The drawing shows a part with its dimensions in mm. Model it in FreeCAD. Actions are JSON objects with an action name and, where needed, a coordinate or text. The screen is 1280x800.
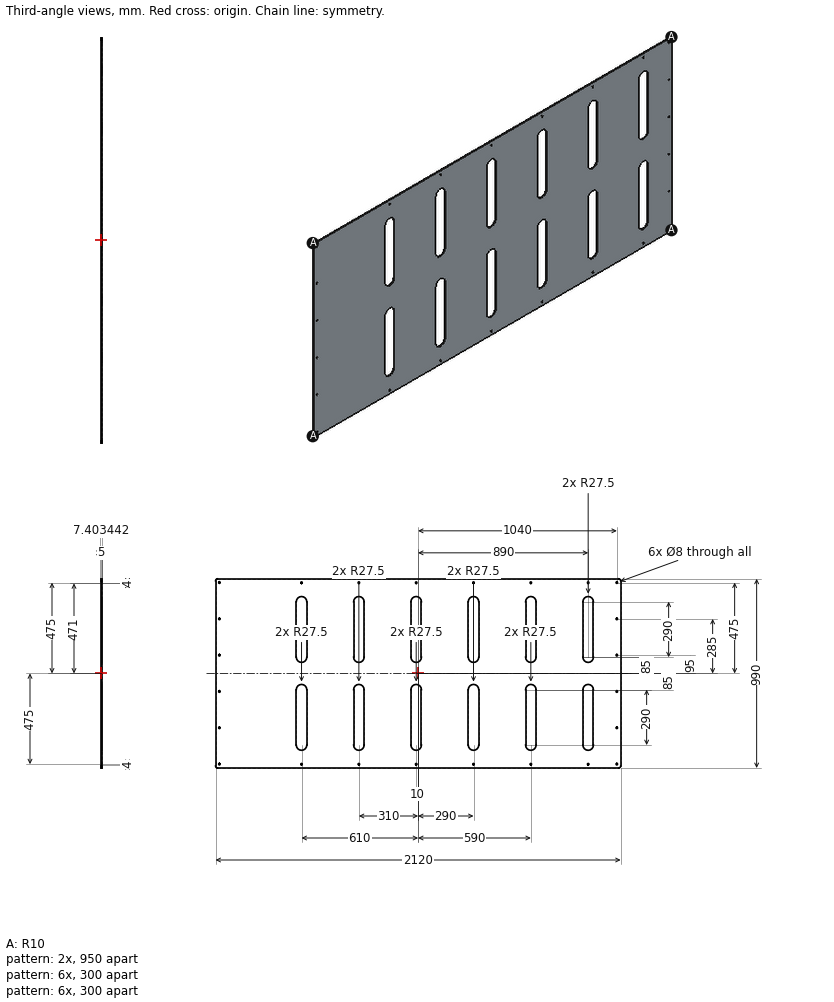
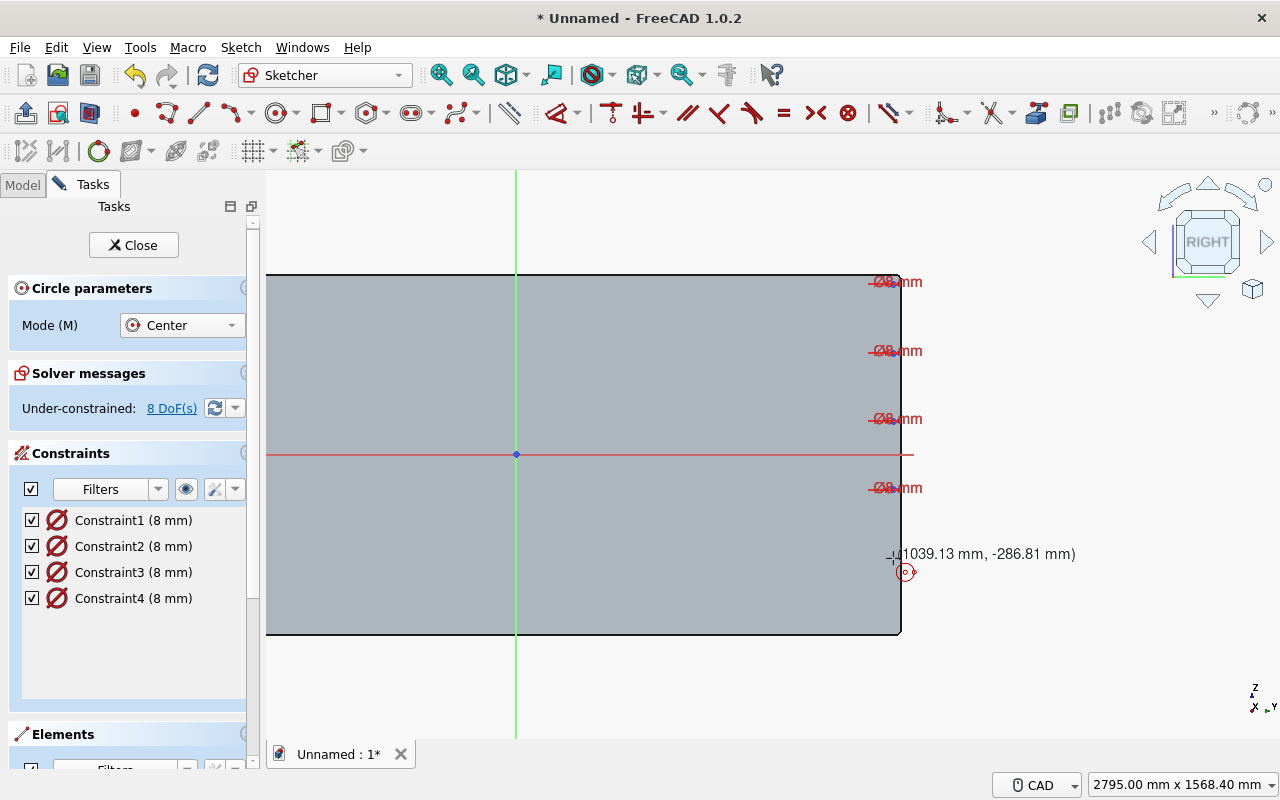
{"action": "left_click", "coordinate": [893, 558]}
{"action": "mouse_move", "coordinate": [894, 557]}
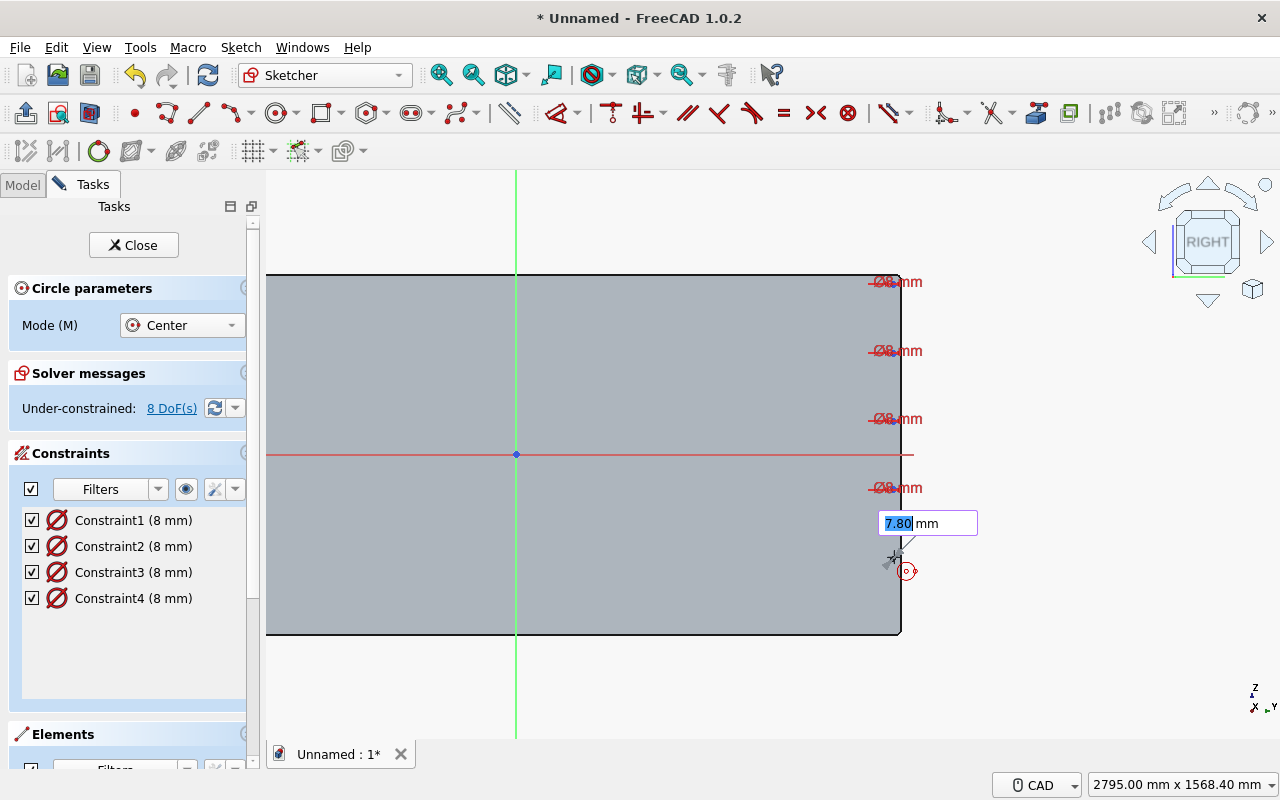
{"action": "type", "text": "8"}
{"action": "key", "text": "Return"}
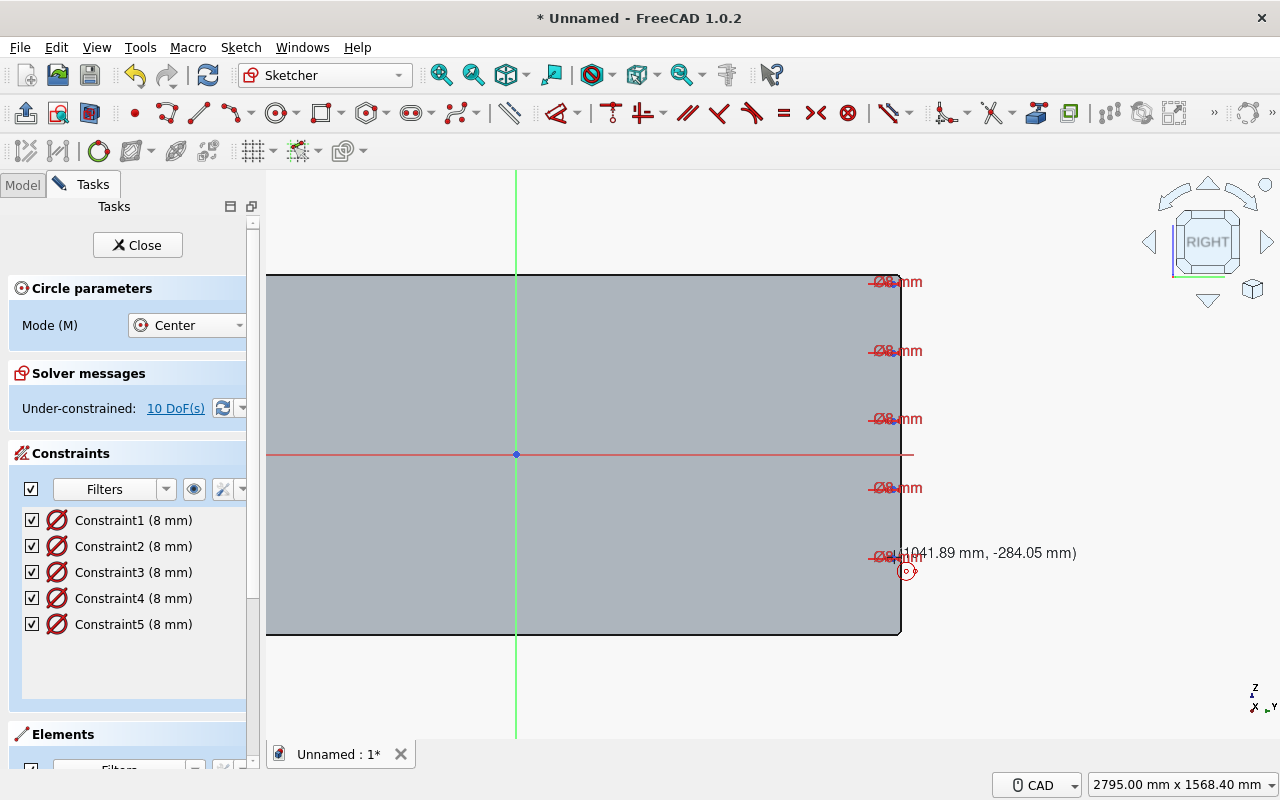
{"action": "scroll", "coordinate": [893, 627], "scroll_direction": "up", "scroll_amount": 14}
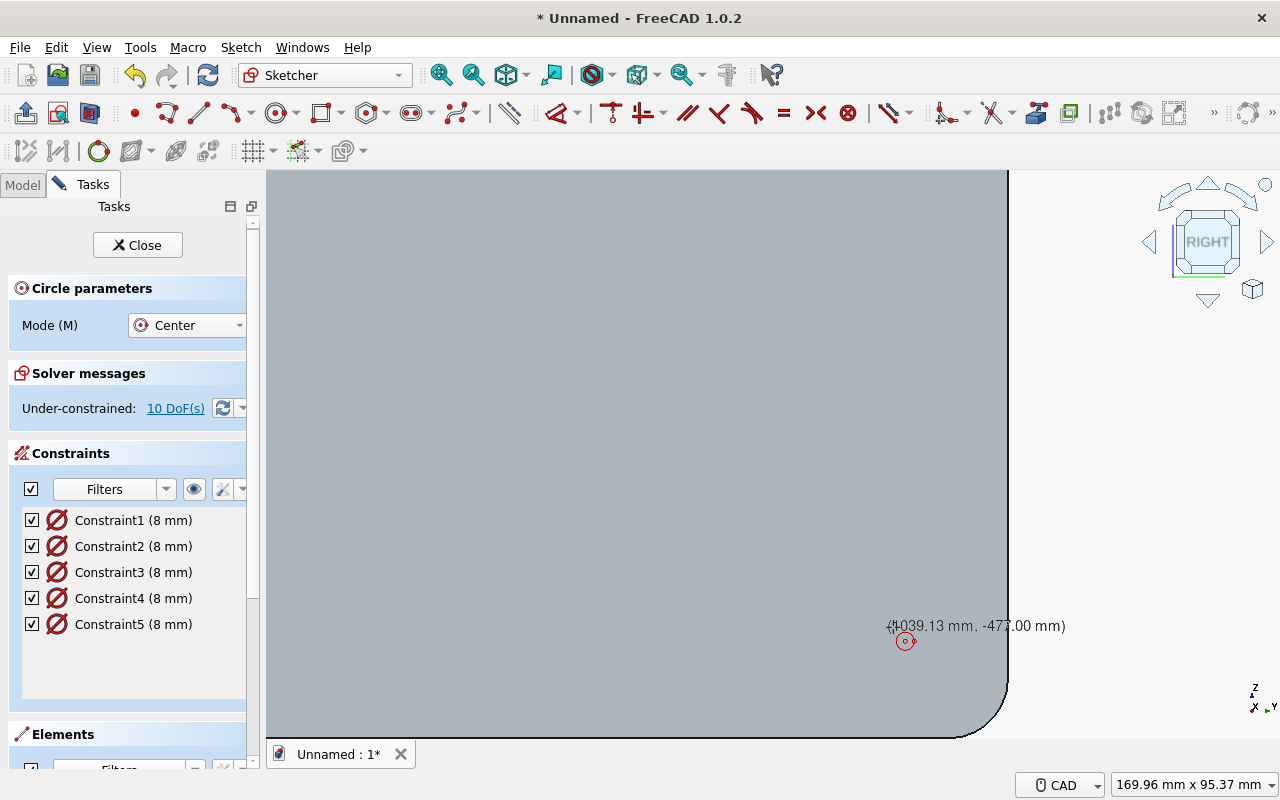
{"action": "scroll", "coordinate": [893, 627], "scroll_direction": "down", "scroll_amount": 14}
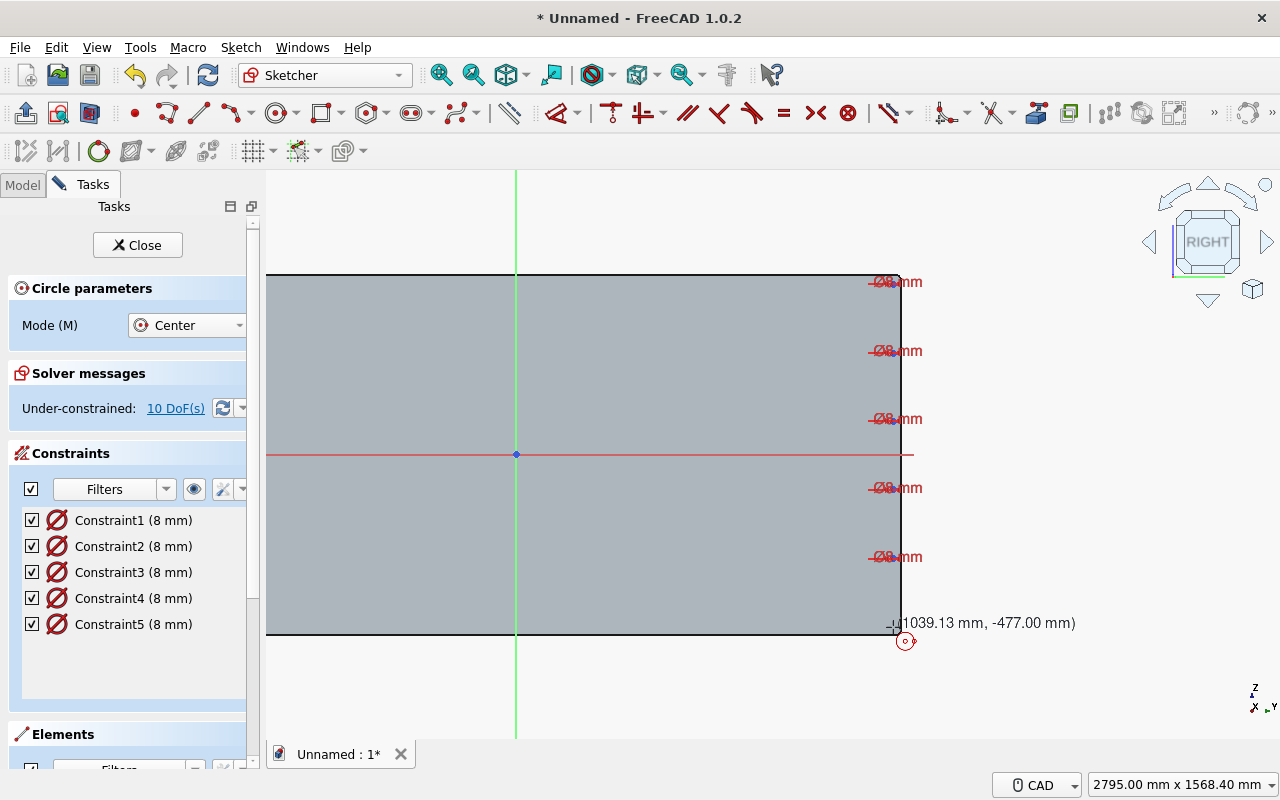
{"action": "left_click", "coordinate": [893, 627]}
{"action": "mouse_move", "coordinate": [894, 626]}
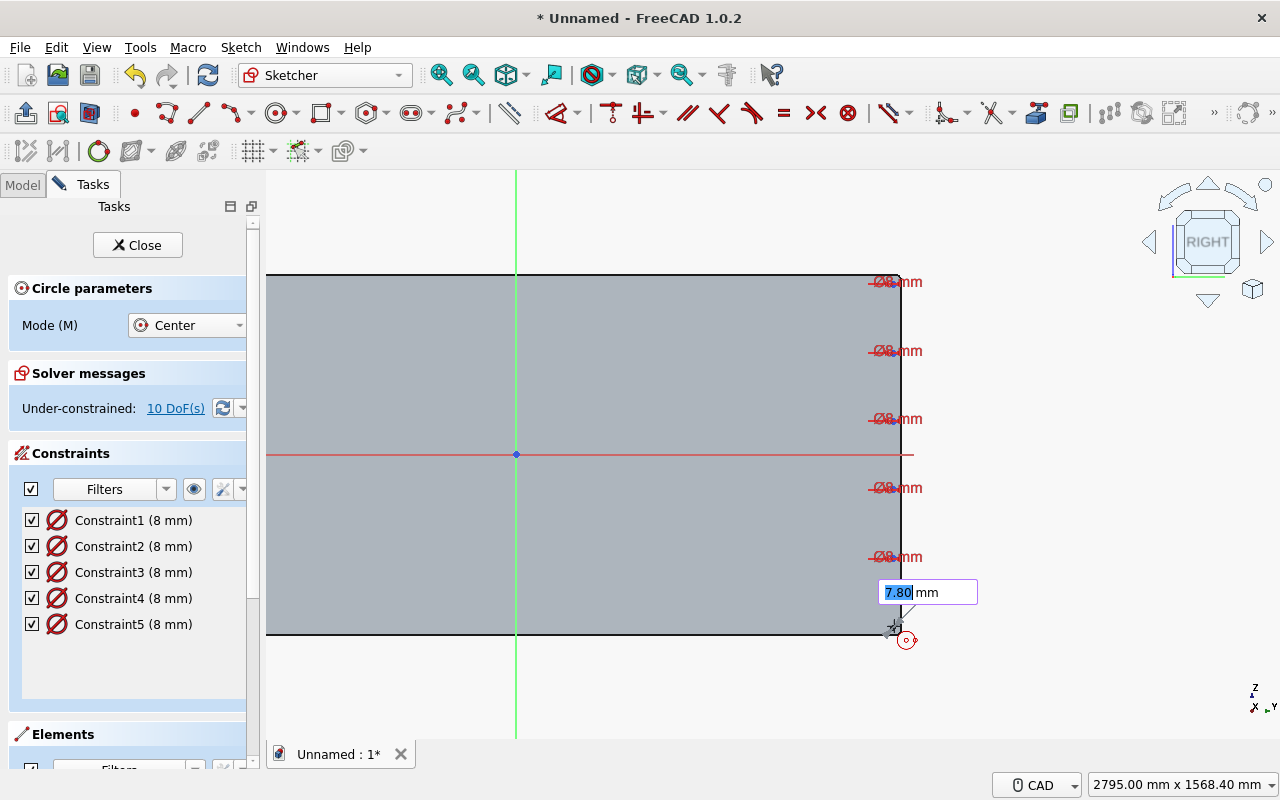
{"action": "type", "text": "8"}
{"action": "key", "text": "Return"}
{"action": "key", "text": "Escape"}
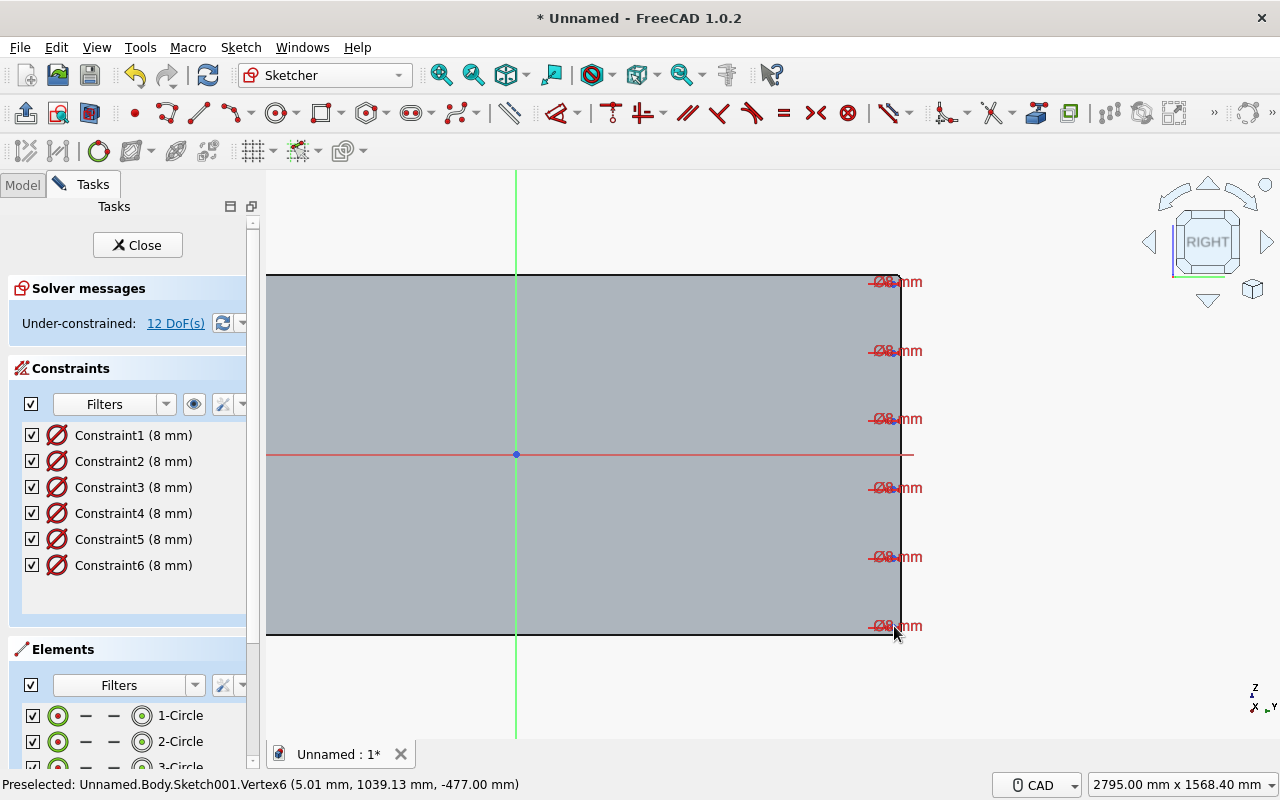
{"action": "left_click", "coordinate": [893, 421]}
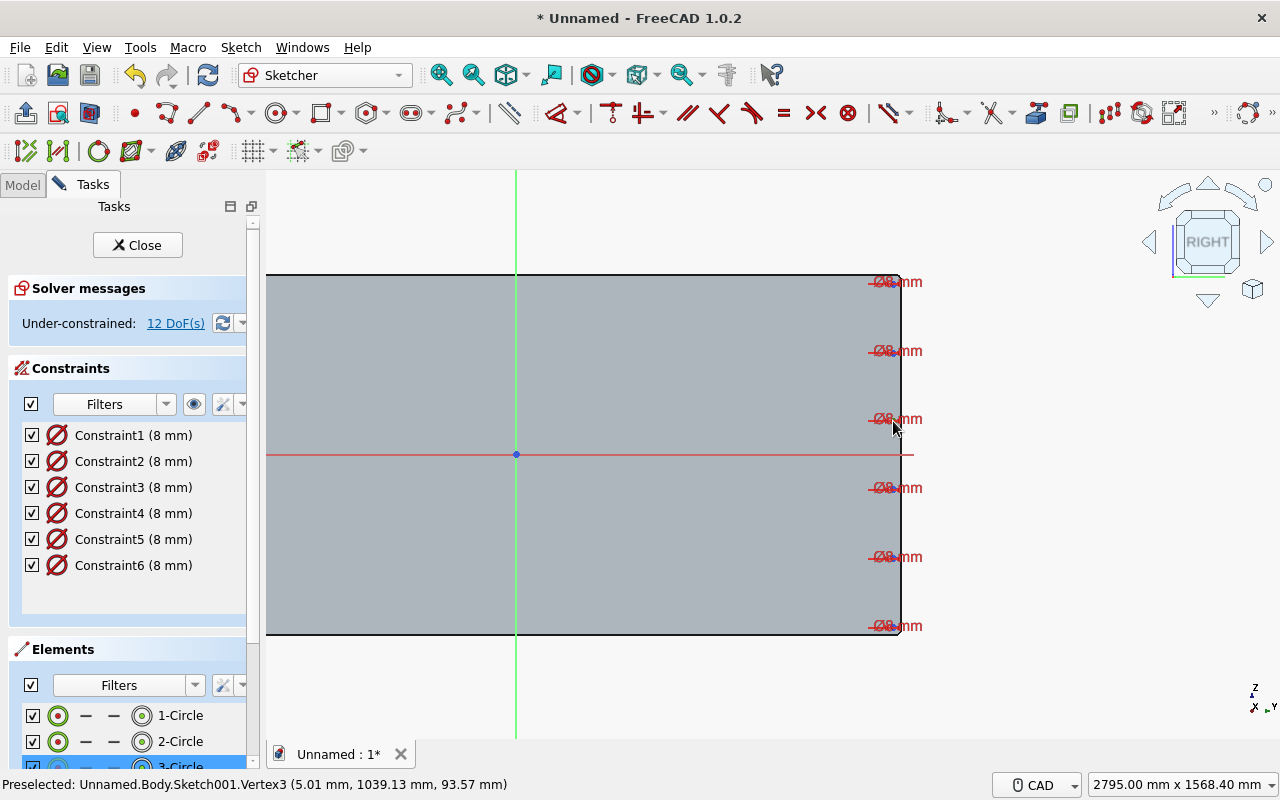
{"action": "left_click", "coordinate": [893, 490]}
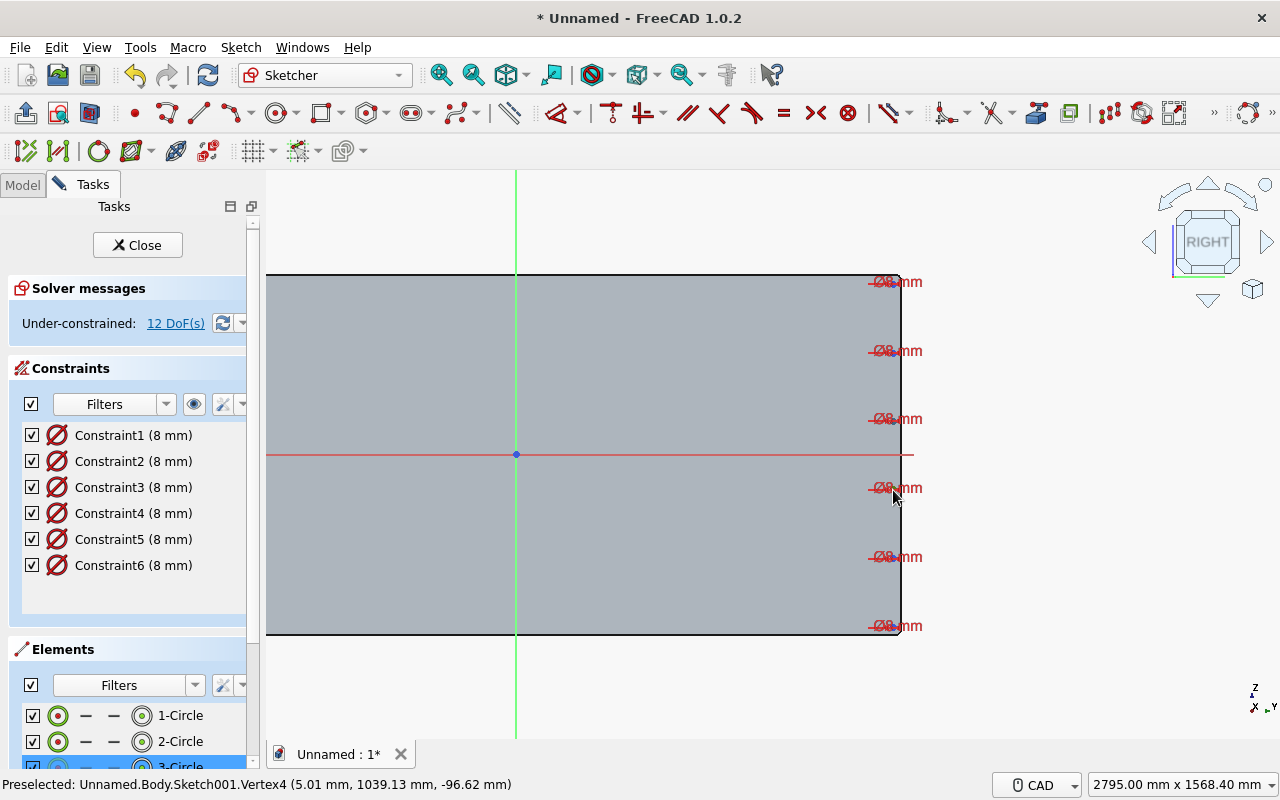
{"action": "left_click", "coordinate": [353, 455]}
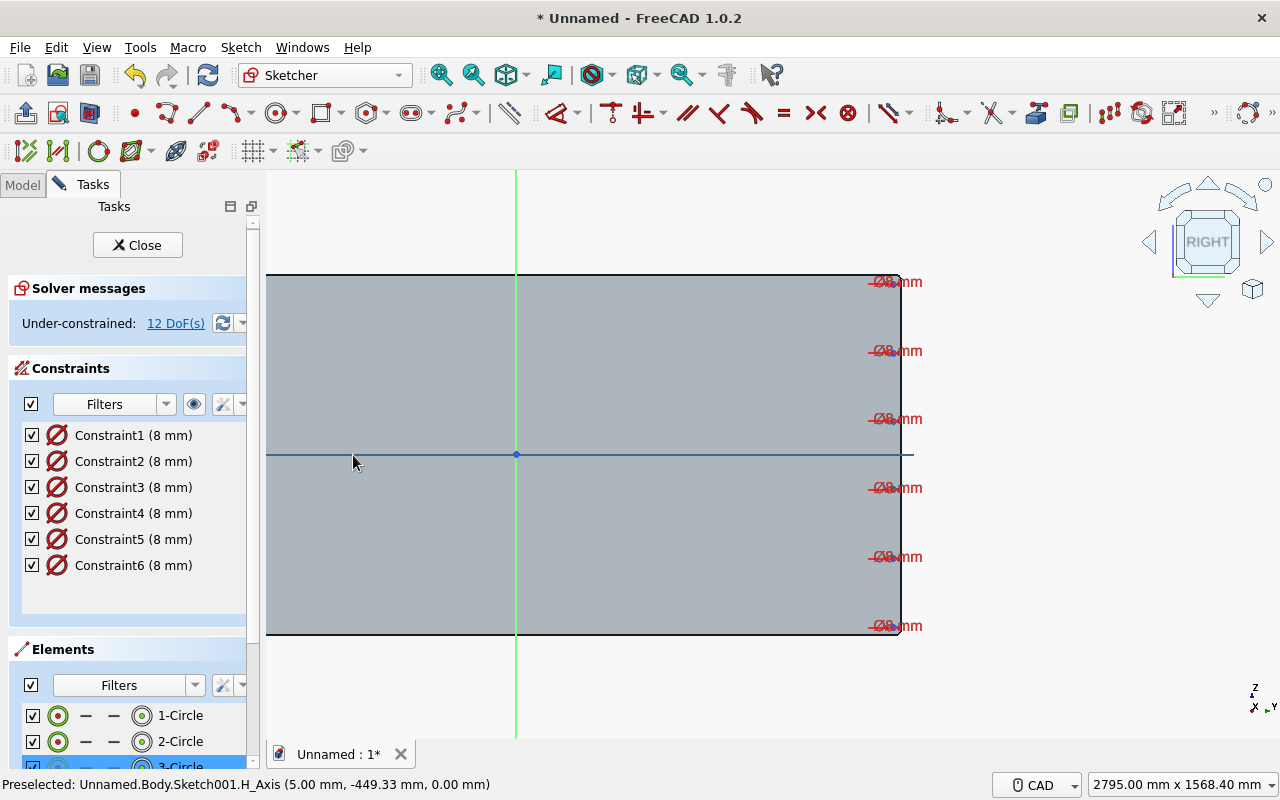
{"action": "key", "text": "s"}